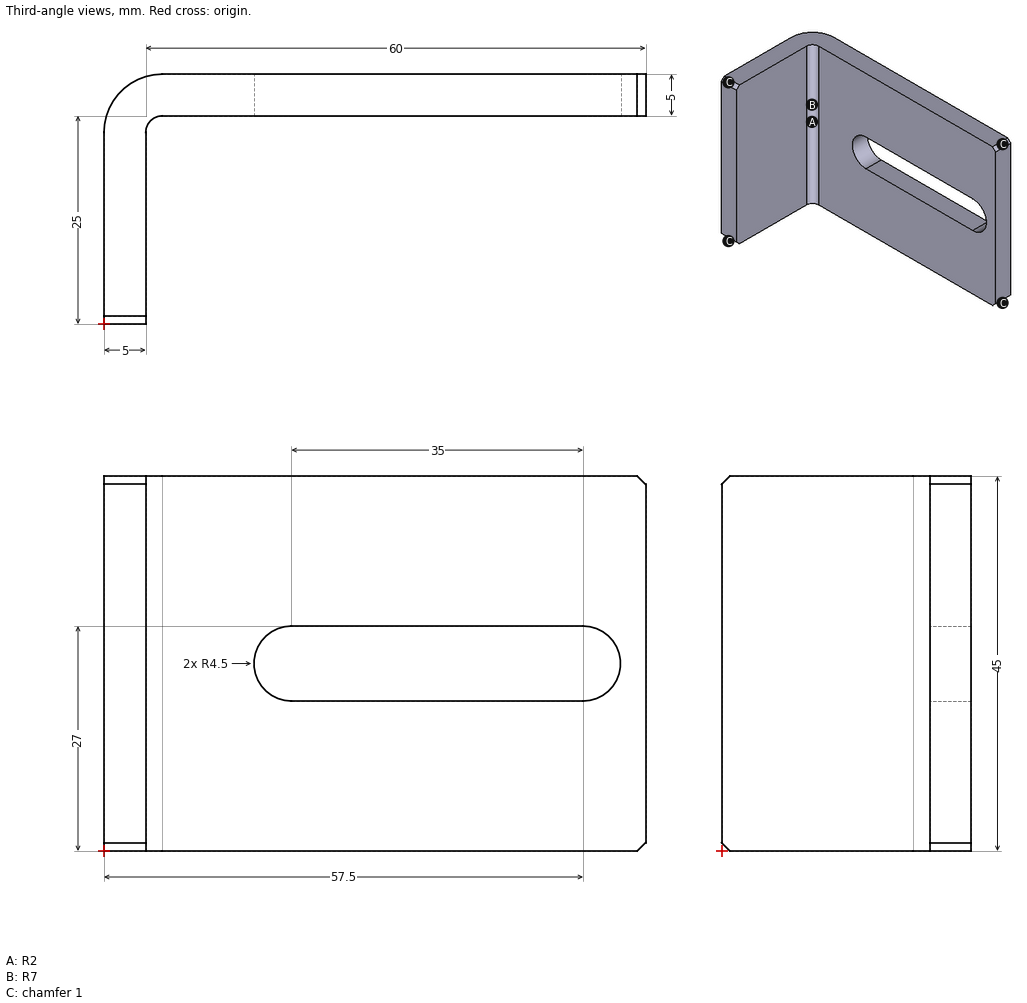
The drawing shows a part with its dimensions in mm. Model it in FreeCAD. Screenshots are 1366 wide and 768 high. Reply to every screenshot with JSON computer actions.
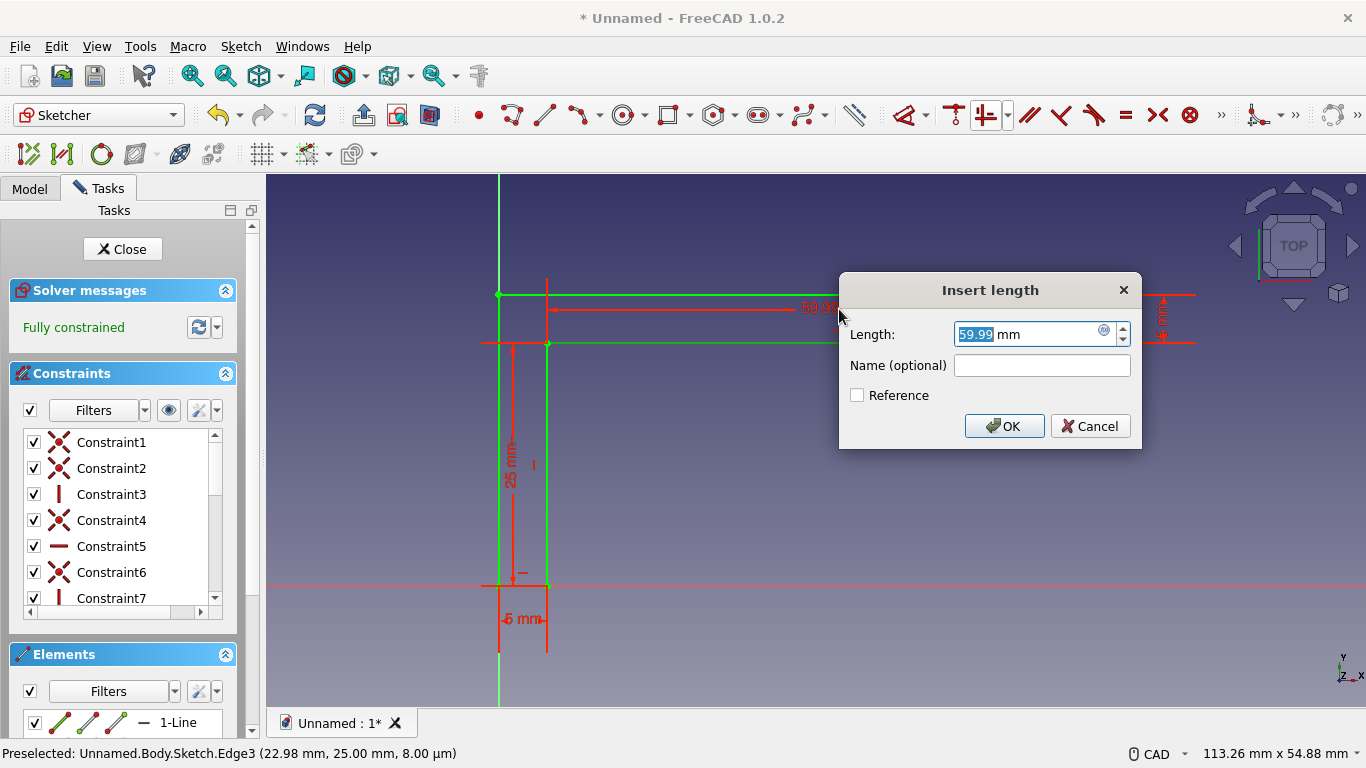
{"action": "type", "text": "60"}
{"action": "key", "text": "Return"}
{"action": "key", "text": "Escape"}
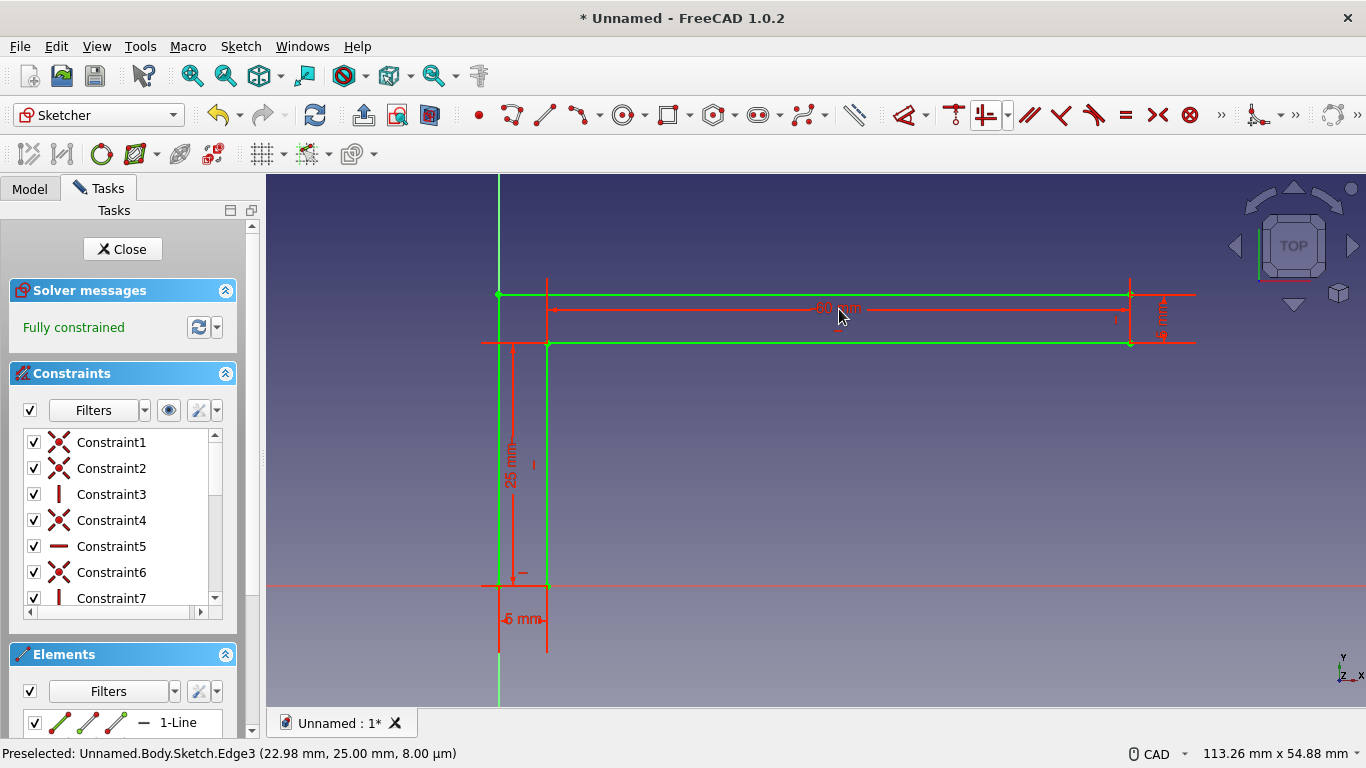
{"action": "left_click", "coordinate": [123, 249]}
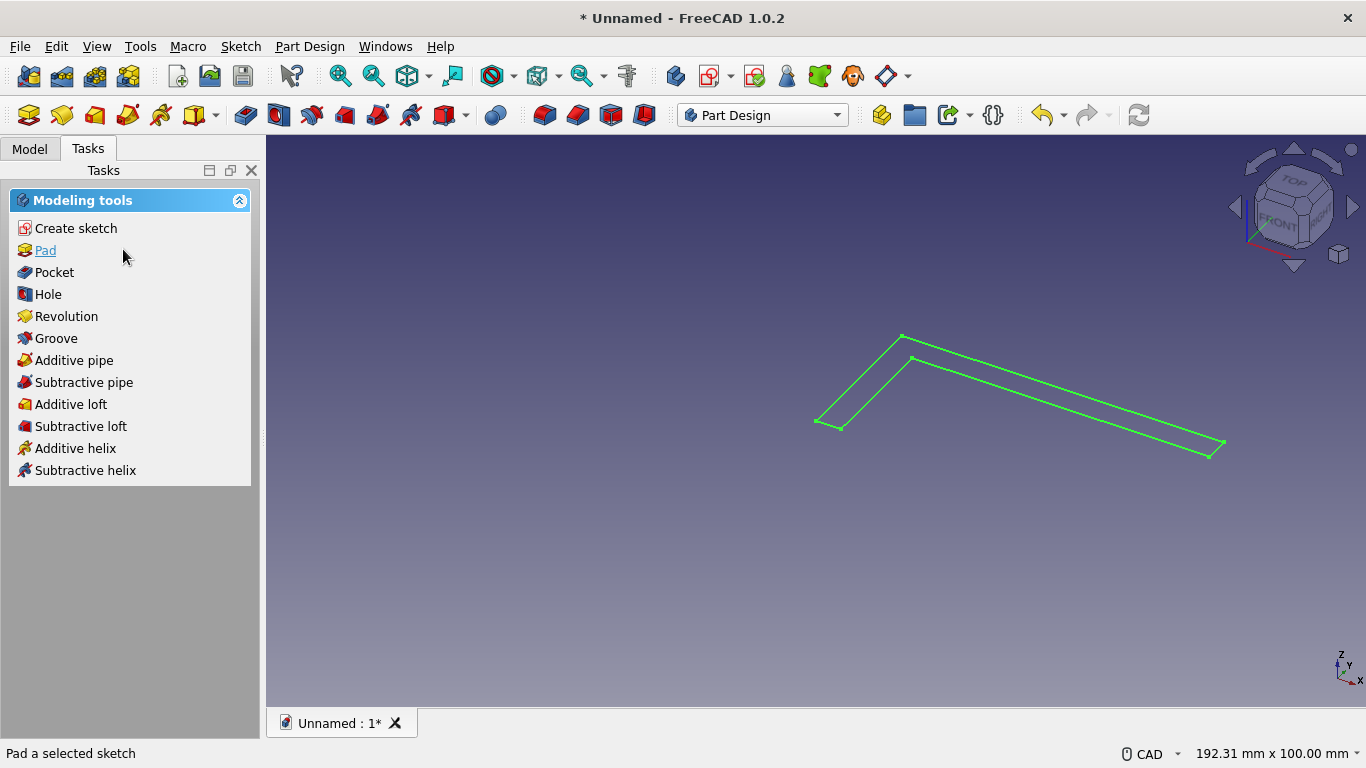
{"action": "left_click", "coordinate": [29, 116]}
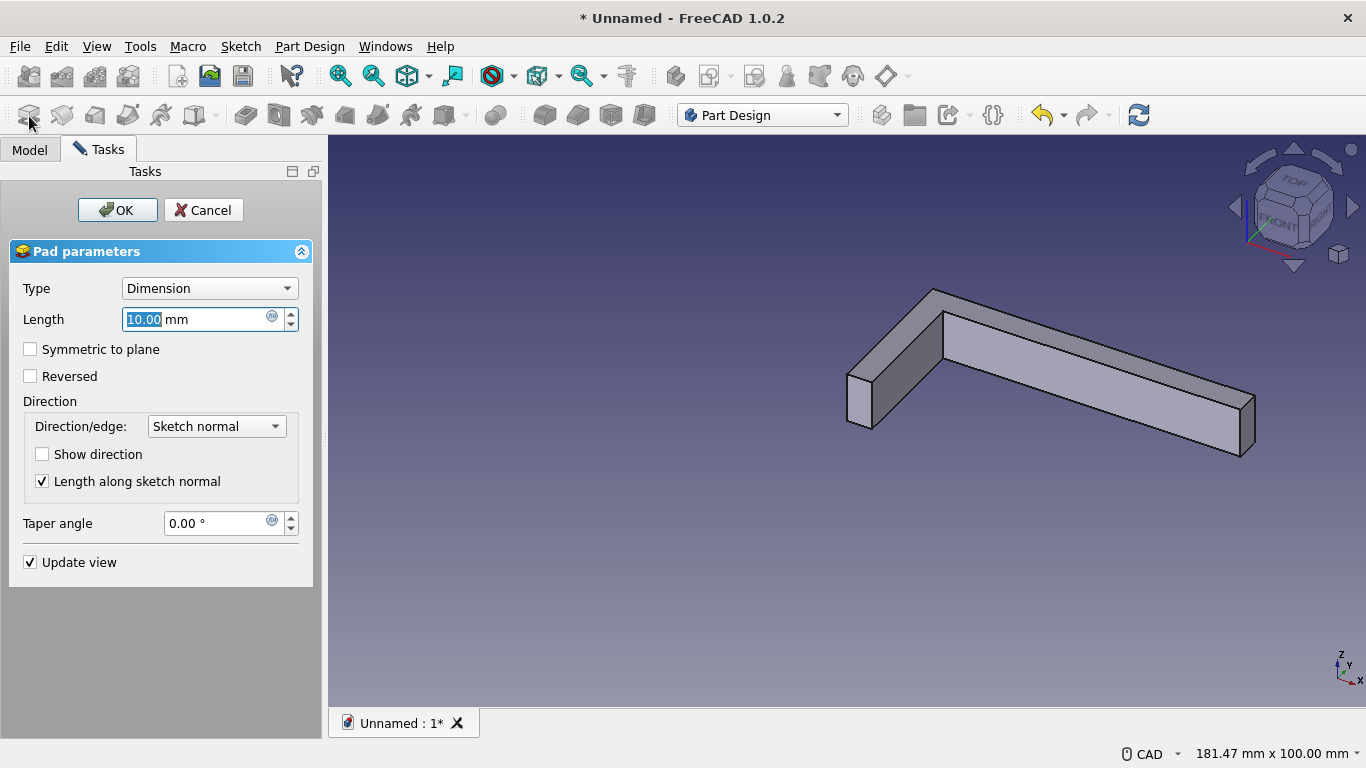
{"action": "type", "text": "45"}
{"action": "key", "text": "Tab"}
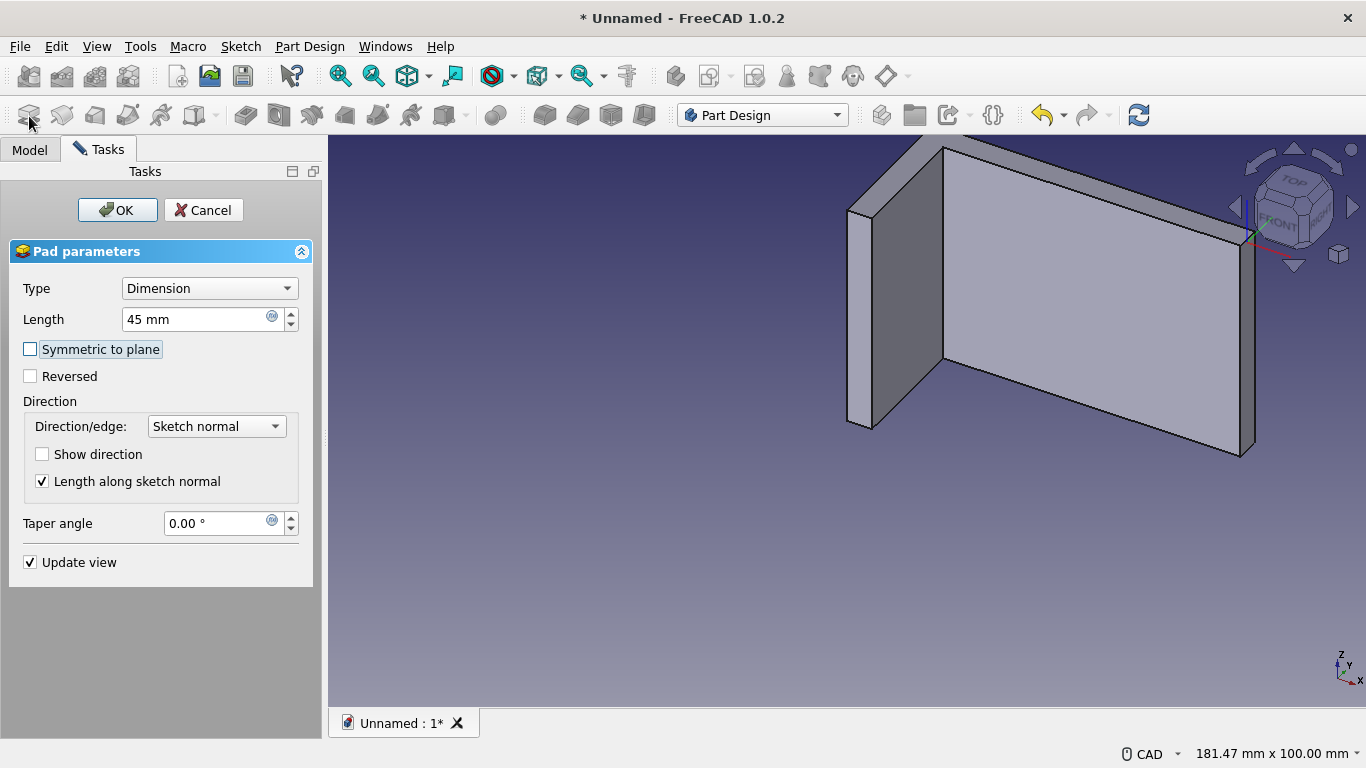
{"action": "left_click", "coordinate": [118, 210]}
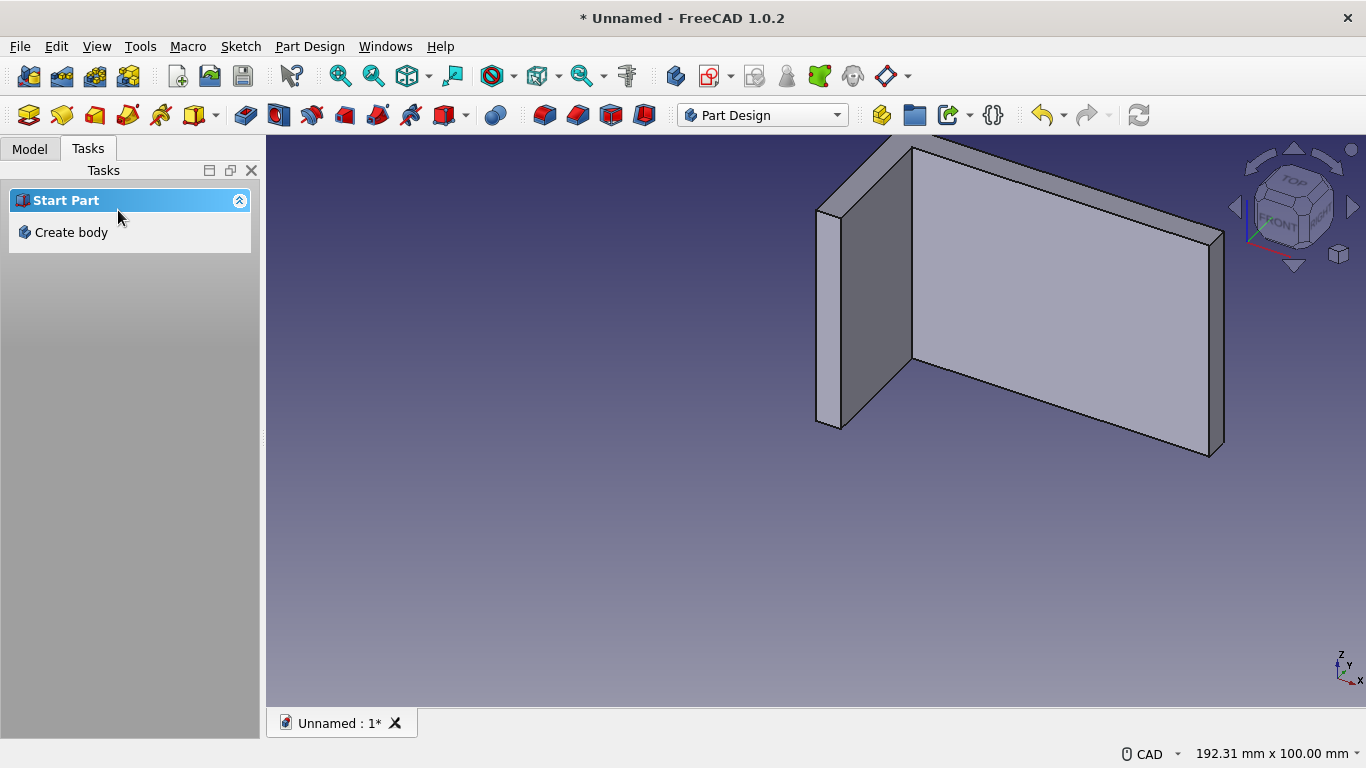
{"action": "left_click", "coordinate": [341, 76]}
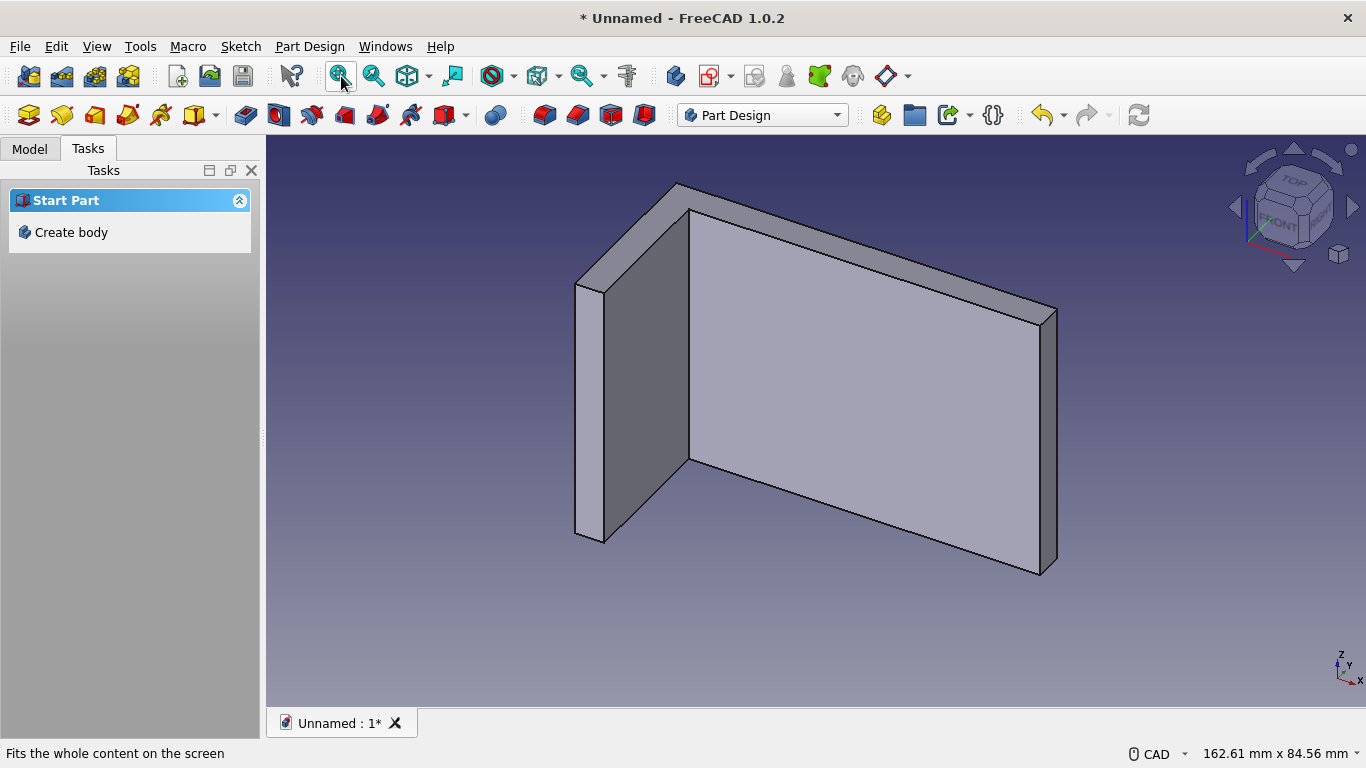
{"action": "key", "text": "0"}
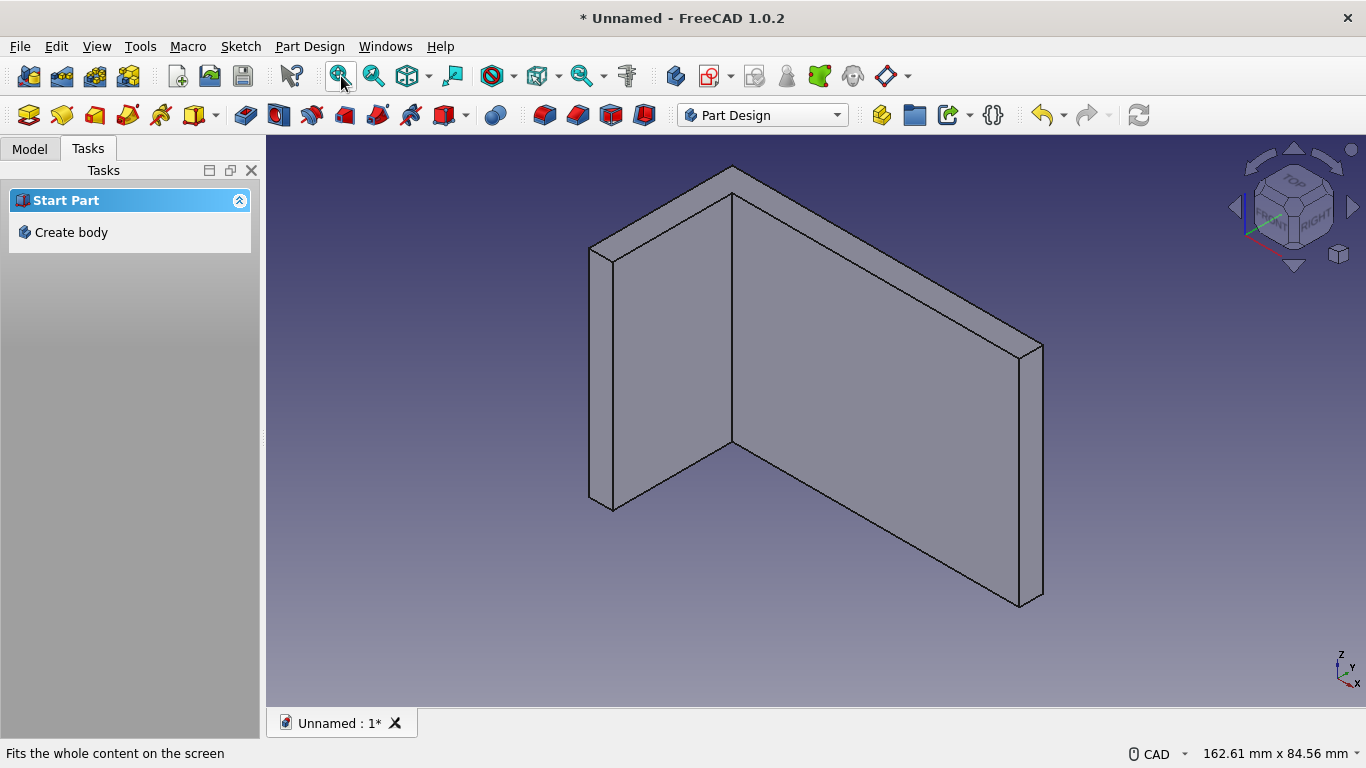
{"action": "key", "text": "2"}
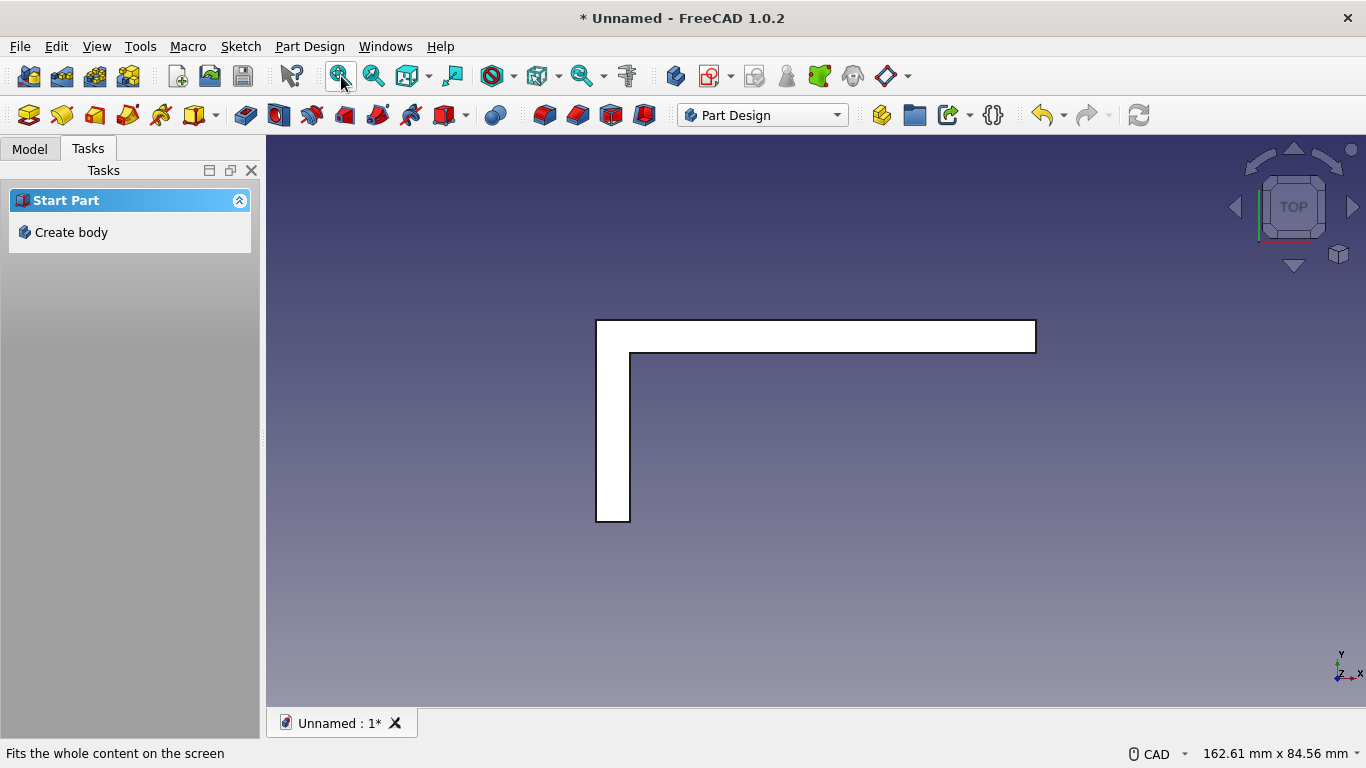
{"action": "left_click", "coordinate": [341, 76]}